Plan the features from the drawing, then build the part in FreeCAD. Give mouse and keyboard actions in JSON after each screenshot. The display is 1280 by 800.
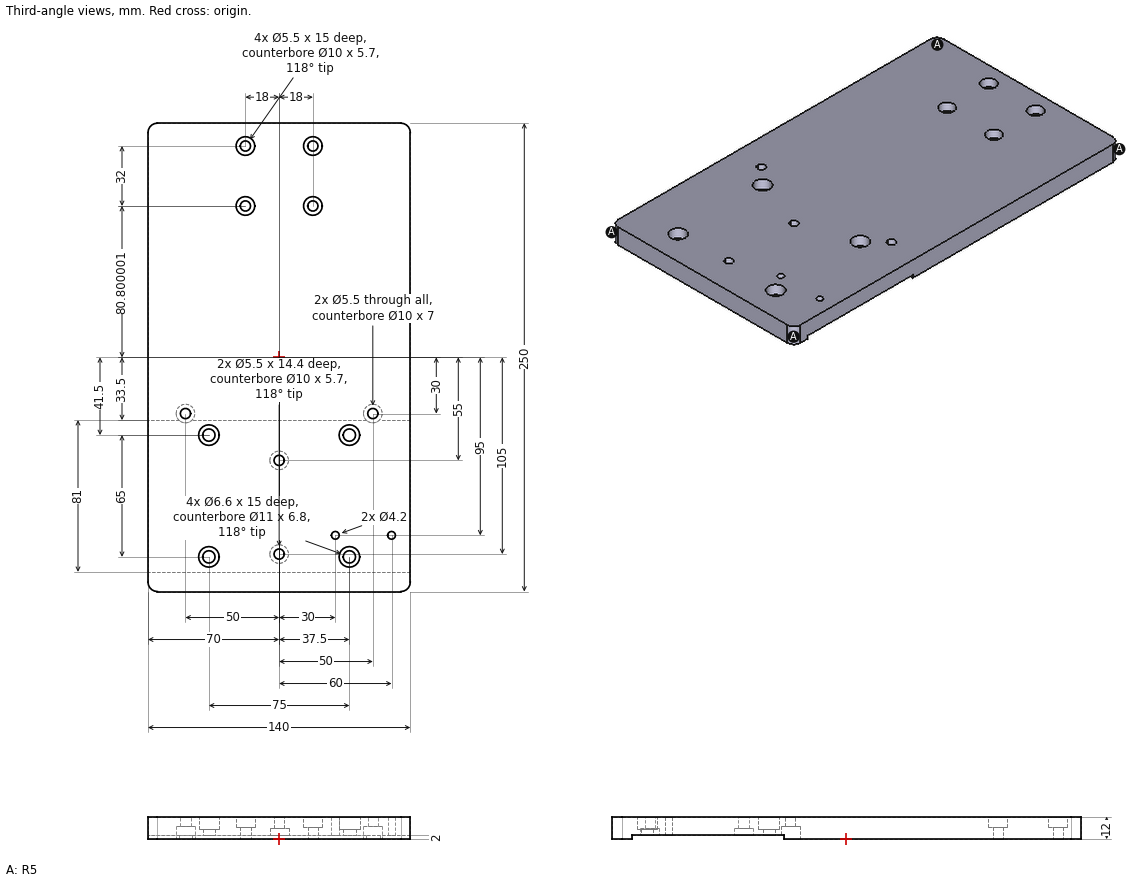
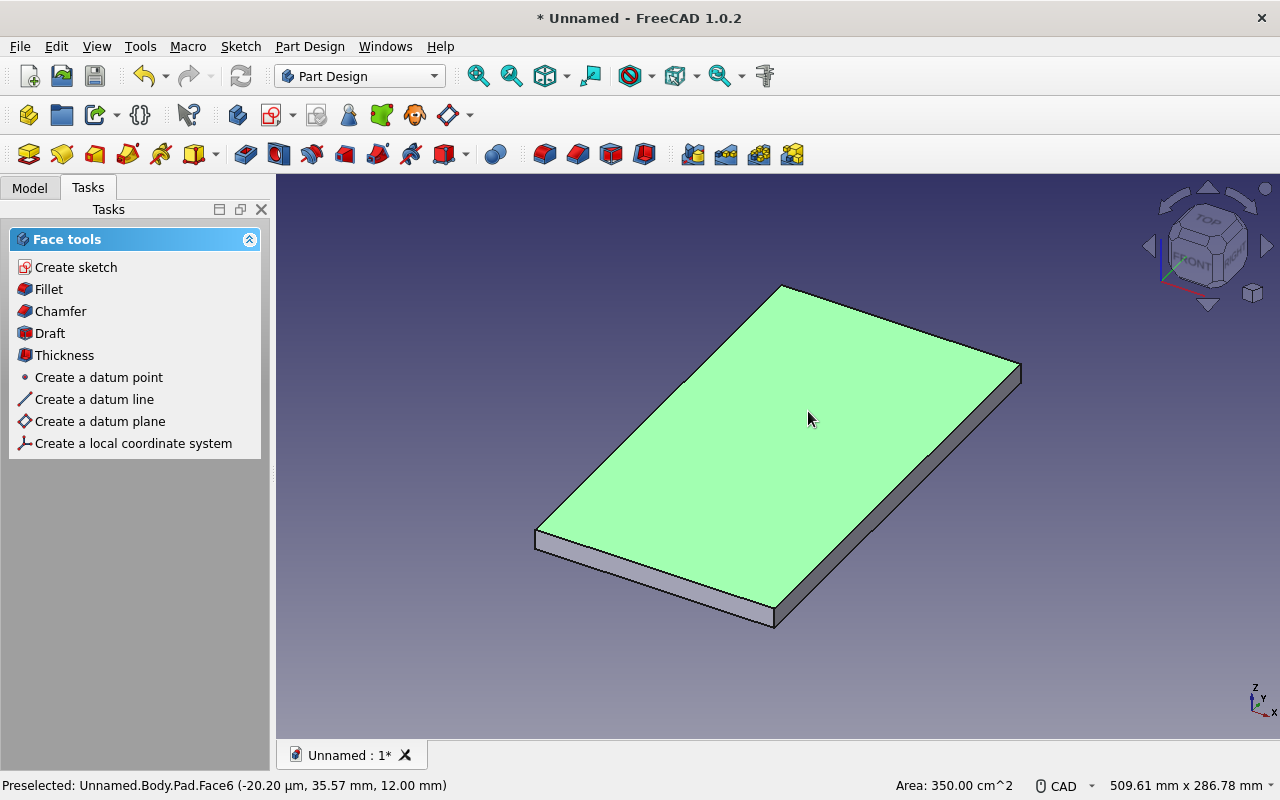
{"action": "left_click", "coordinate": [270, 116]}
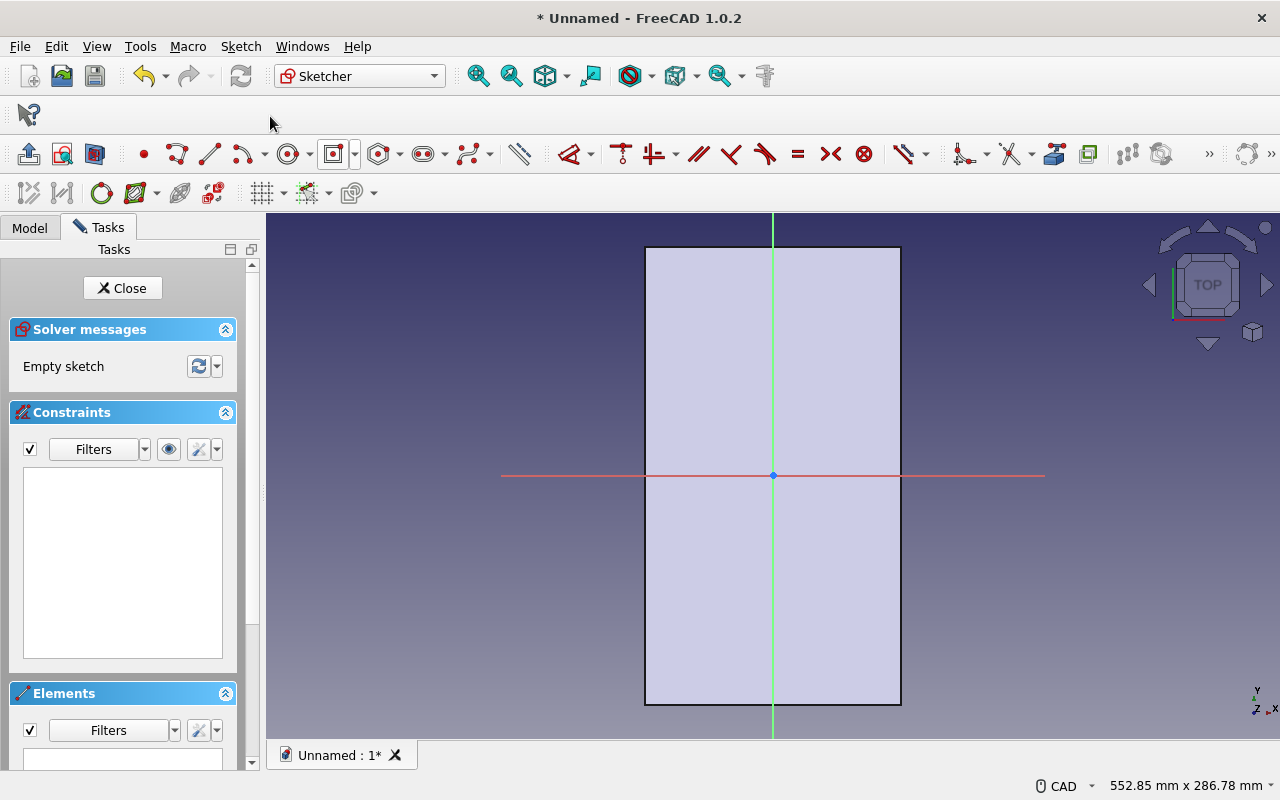
{"action": "scroll", "coordinate": [790, 254], "scroll_direction": "up", "scroll_amount": 8}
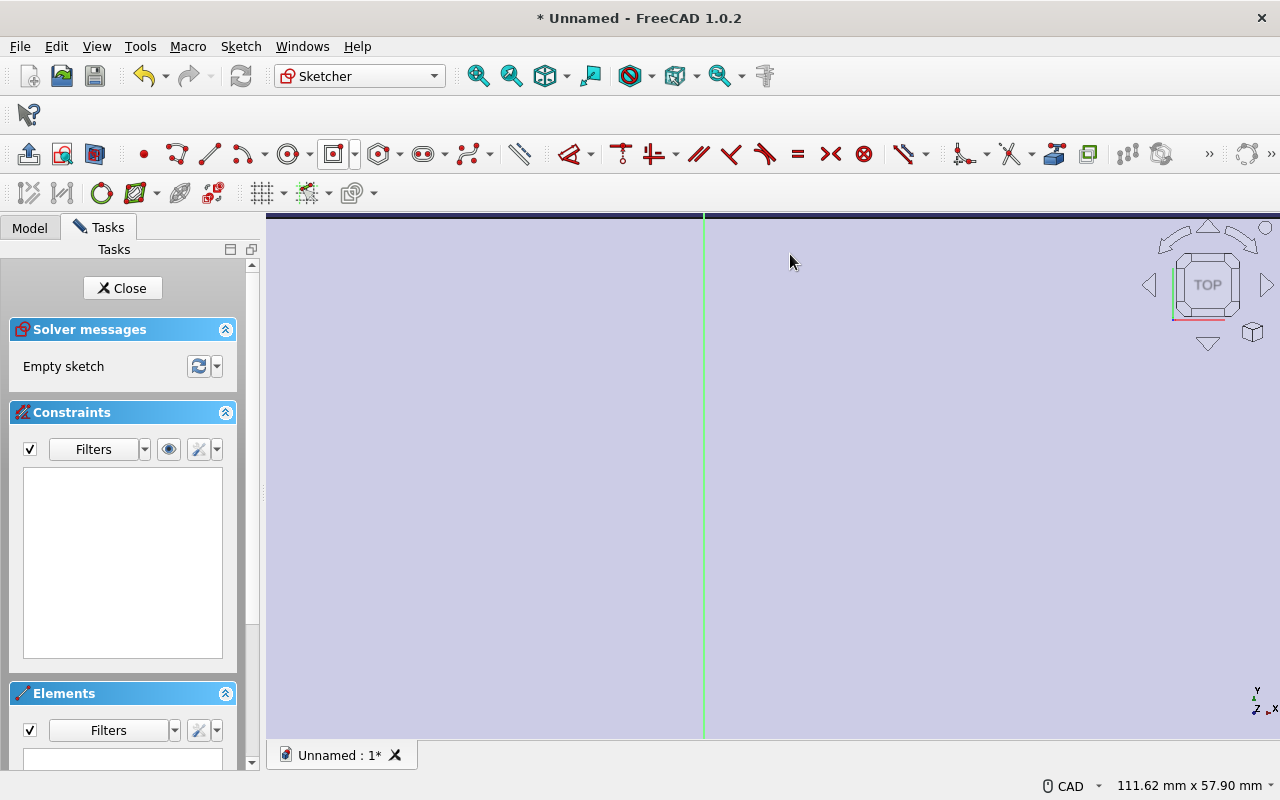
{"action": "left_click", "coordinate": [288, 154]}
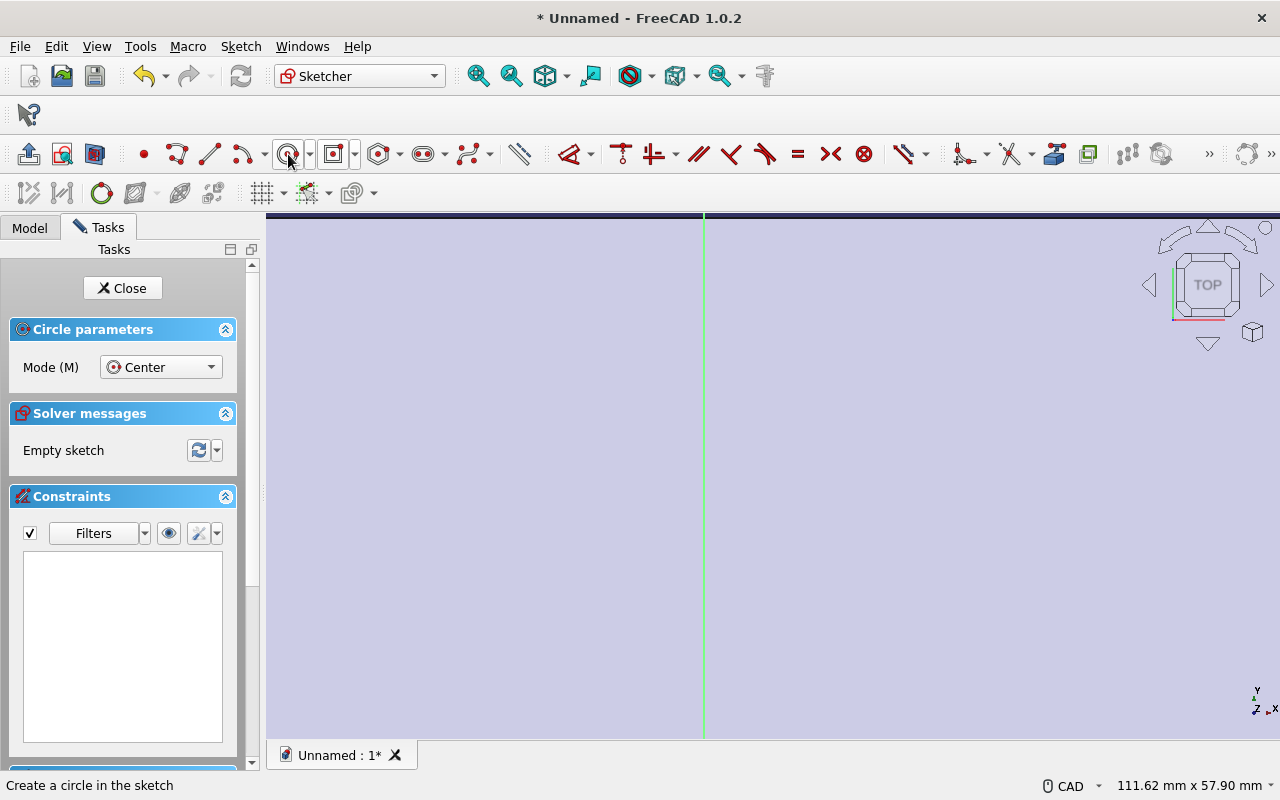
{"action": "left_click", "coordinate": [540, 329]}
{"action": "left_click", "coordinate": [558, 311]}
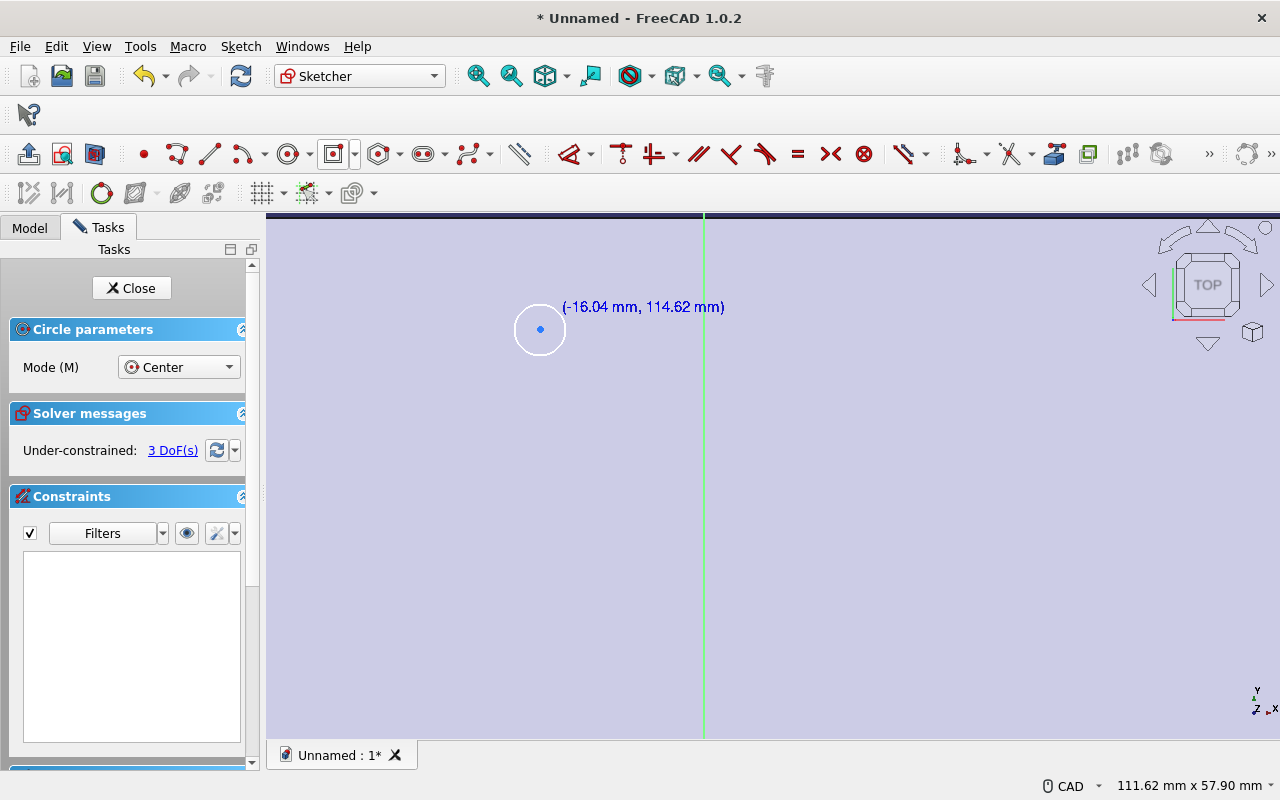
{"action": "left_click", "coordinate": [540, 619]}
{"action": "left_click", "coordinate": [558, 602]}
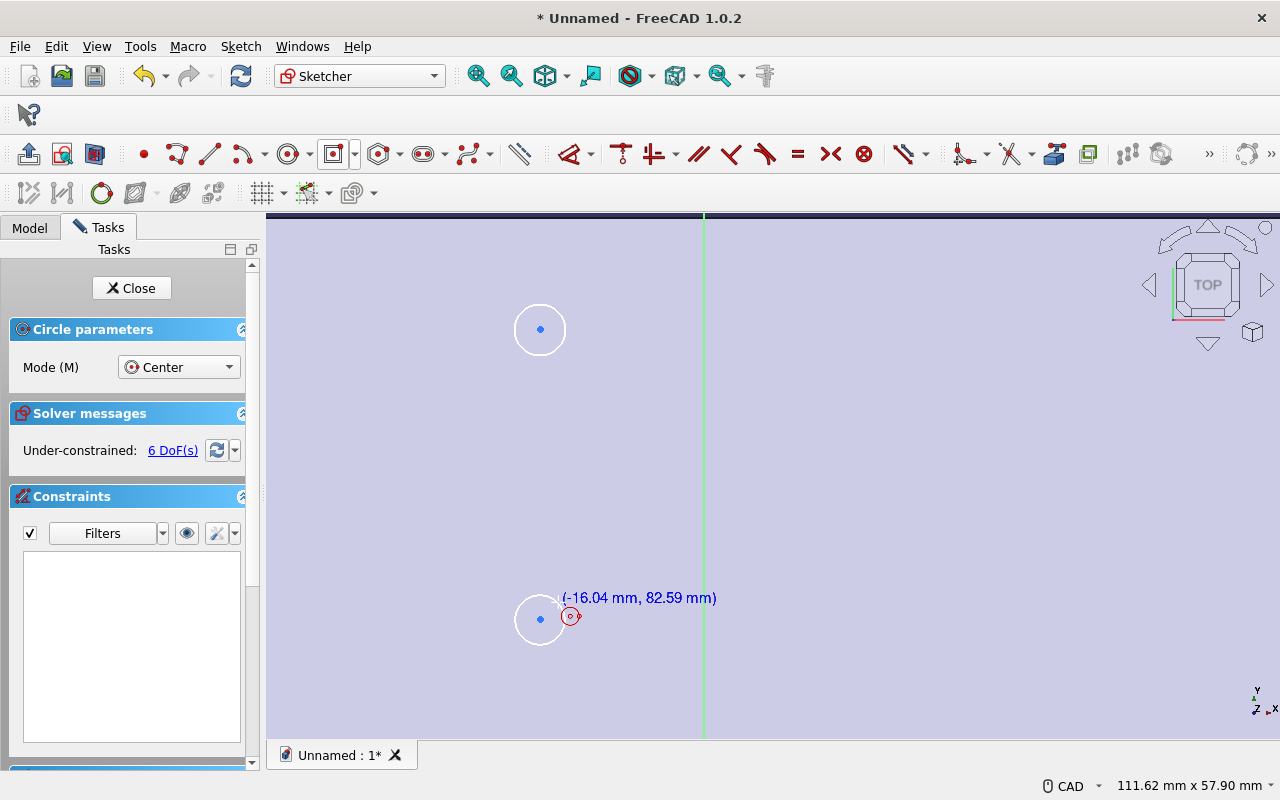
{"action": "left_click", "coordinate": [867, 619]}
{"action": "left_click", "coordinate": [885, 602]}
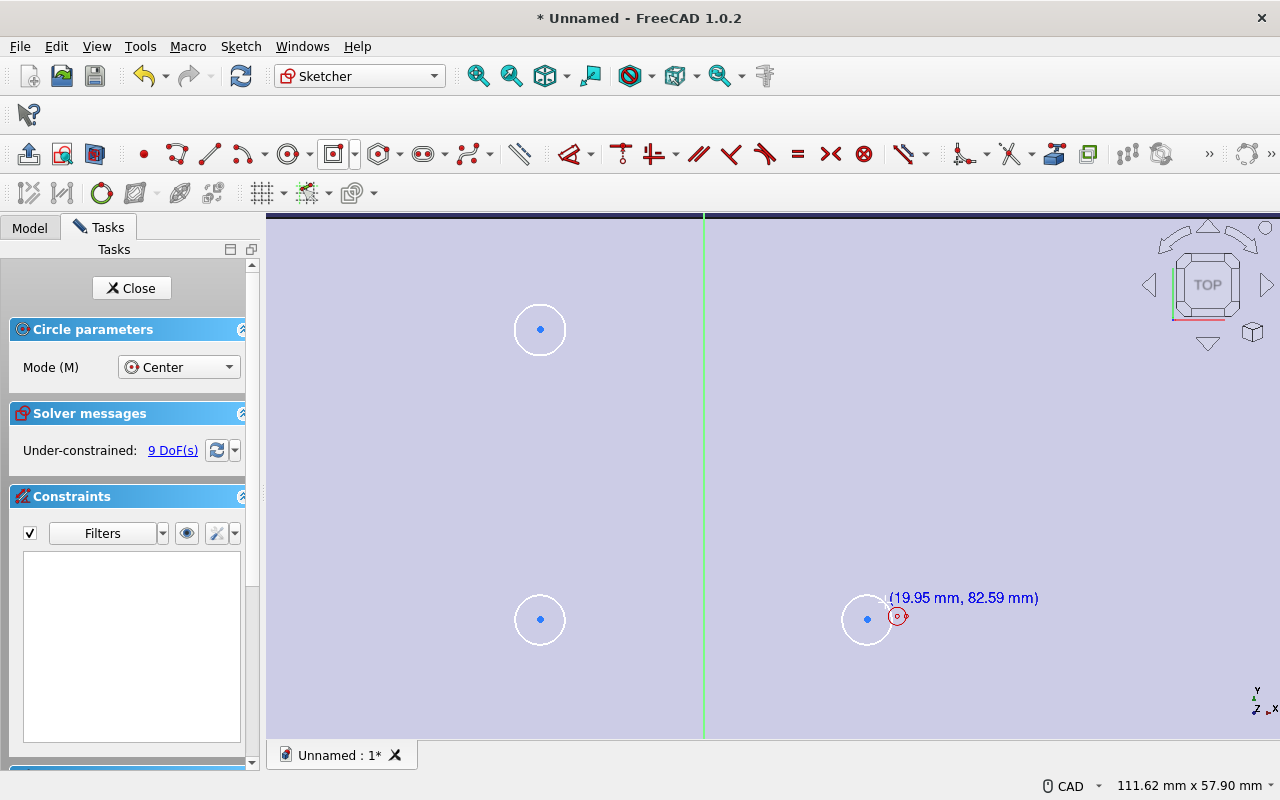
{"action": "left_click", "coordinate": [867, 329]}
{"action": "left_click", "coordinate": [885, 311]}
{"action": "key", "text": "Escape"}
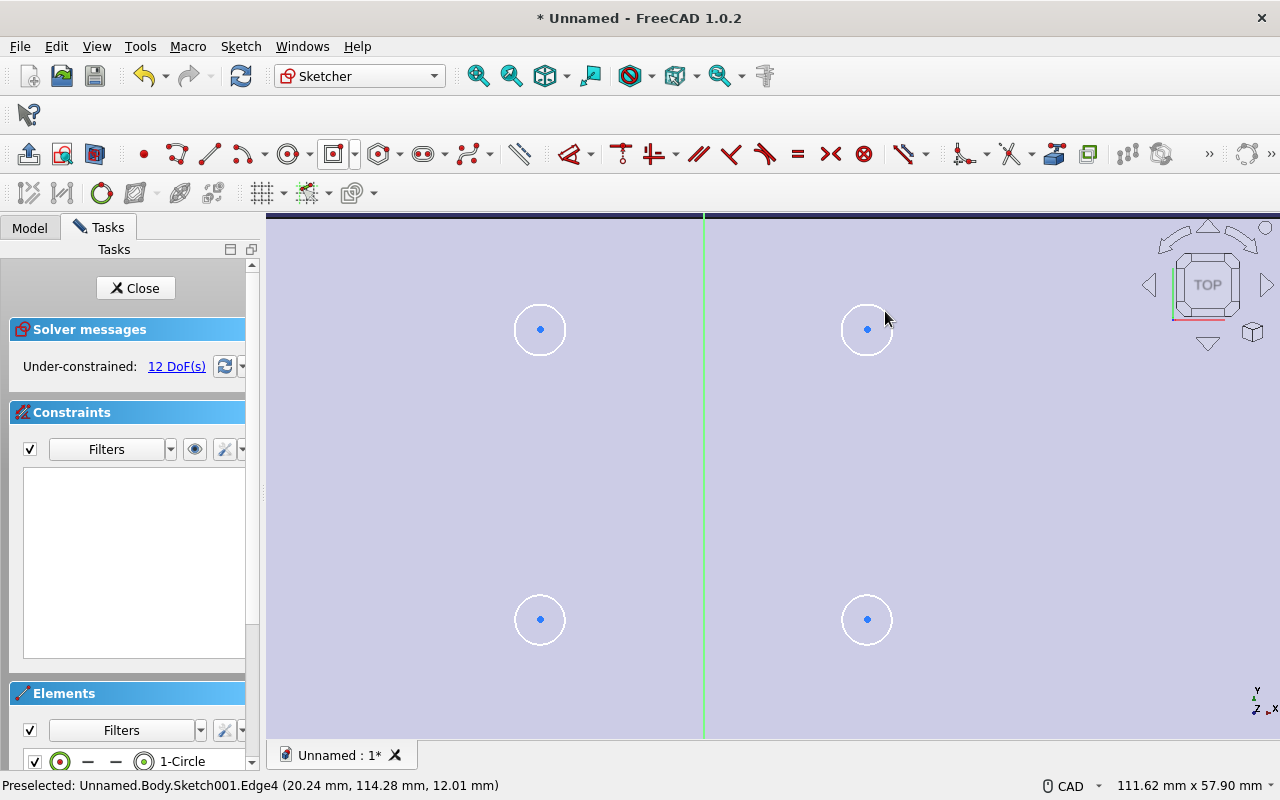
{"action": "left_click", "coordinate": [558, 312]}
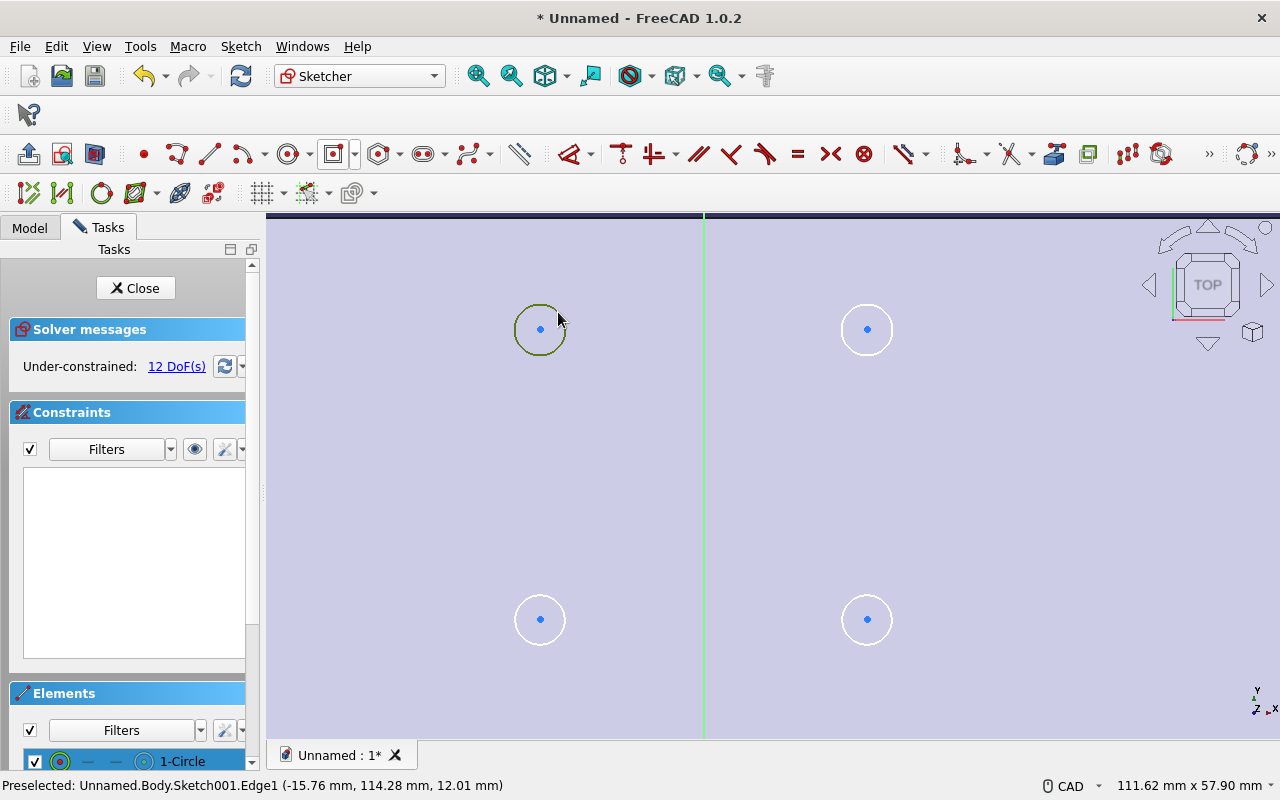
{"action": "left_click", "coordinate": [557, 602]}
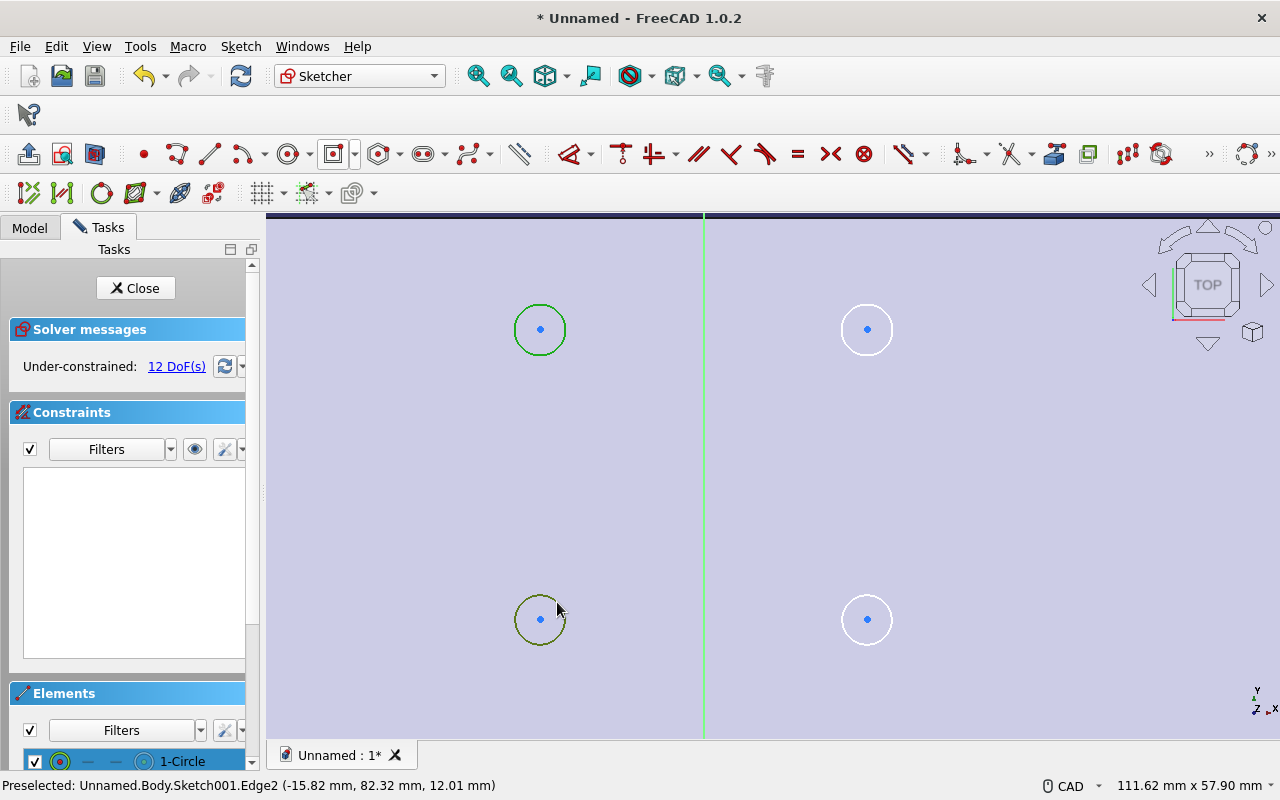
{"action": "left_click", "coordinate": [884, 602]}